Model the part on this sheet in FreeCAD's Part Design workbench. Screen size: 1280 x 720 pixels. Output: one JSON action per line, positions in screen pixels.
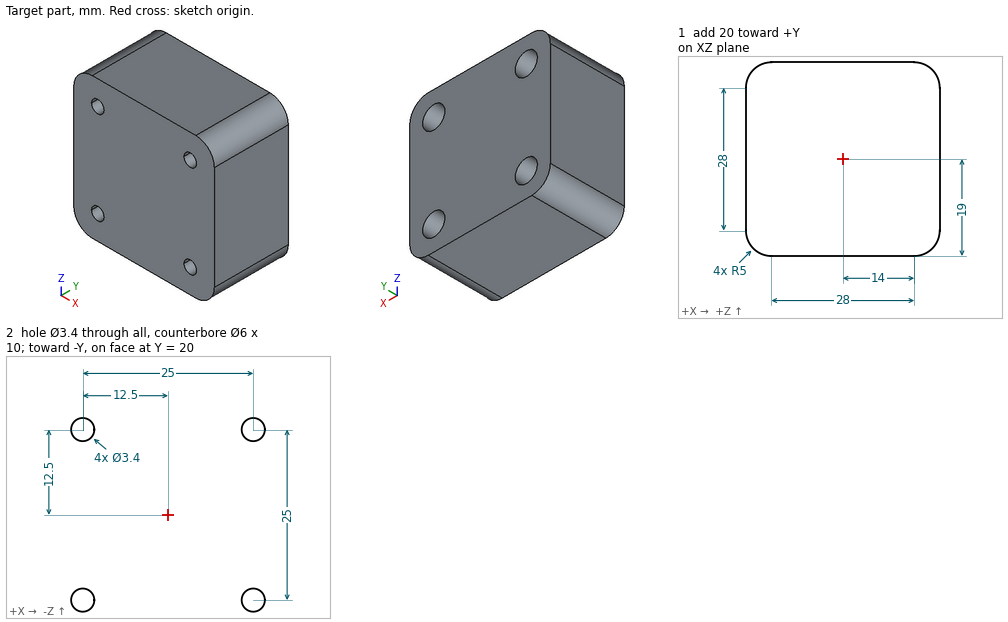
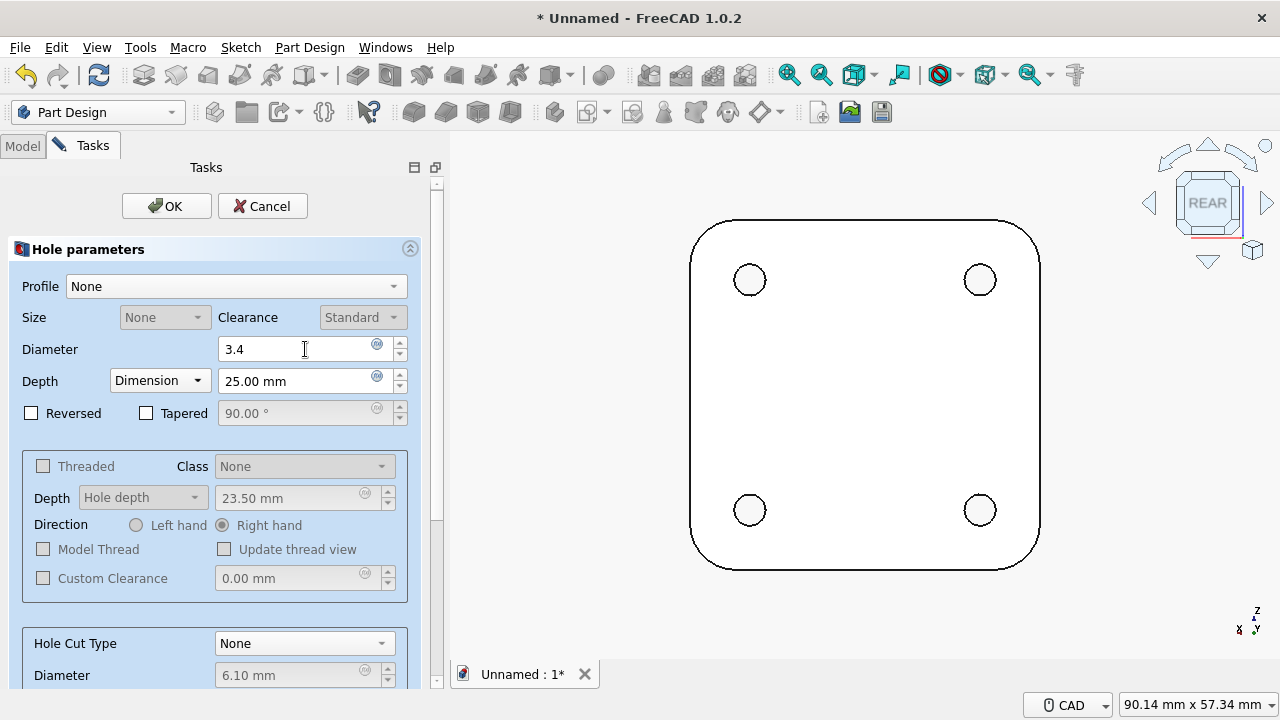
{"action": "left_click", "coordinate": [161, 380]}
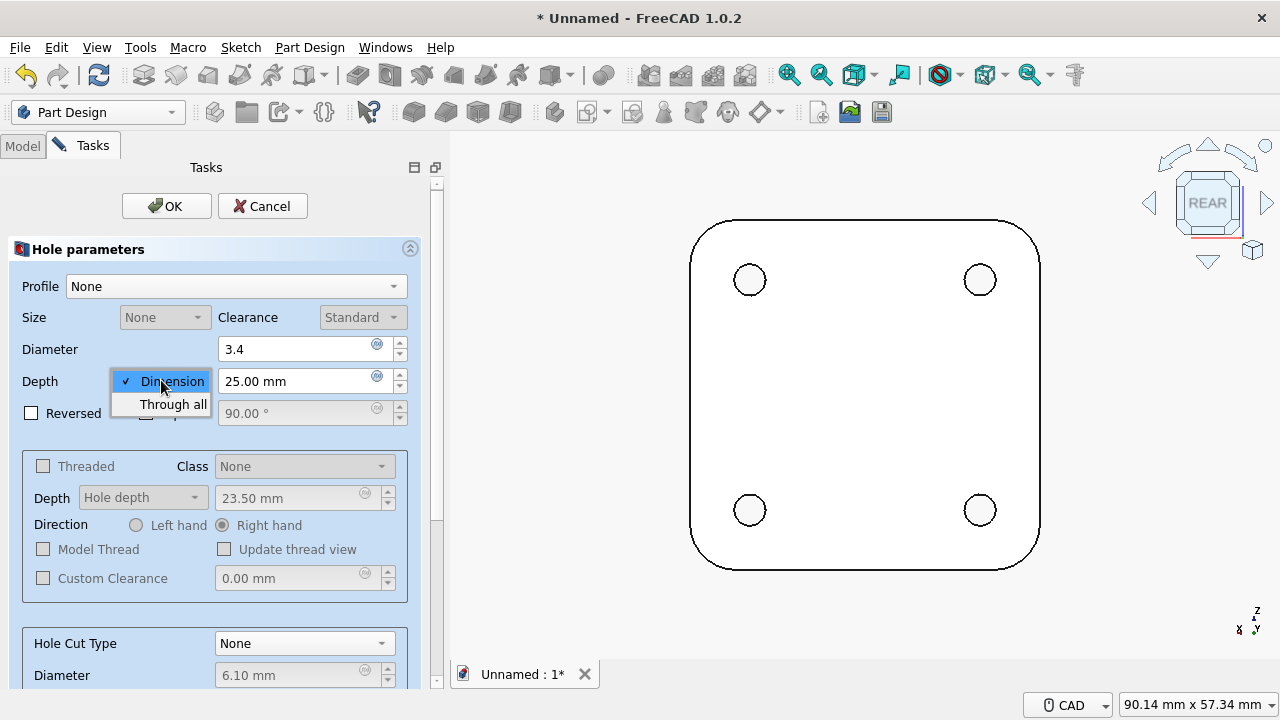
{"action": "left_click", "coordinate": [160, 404]}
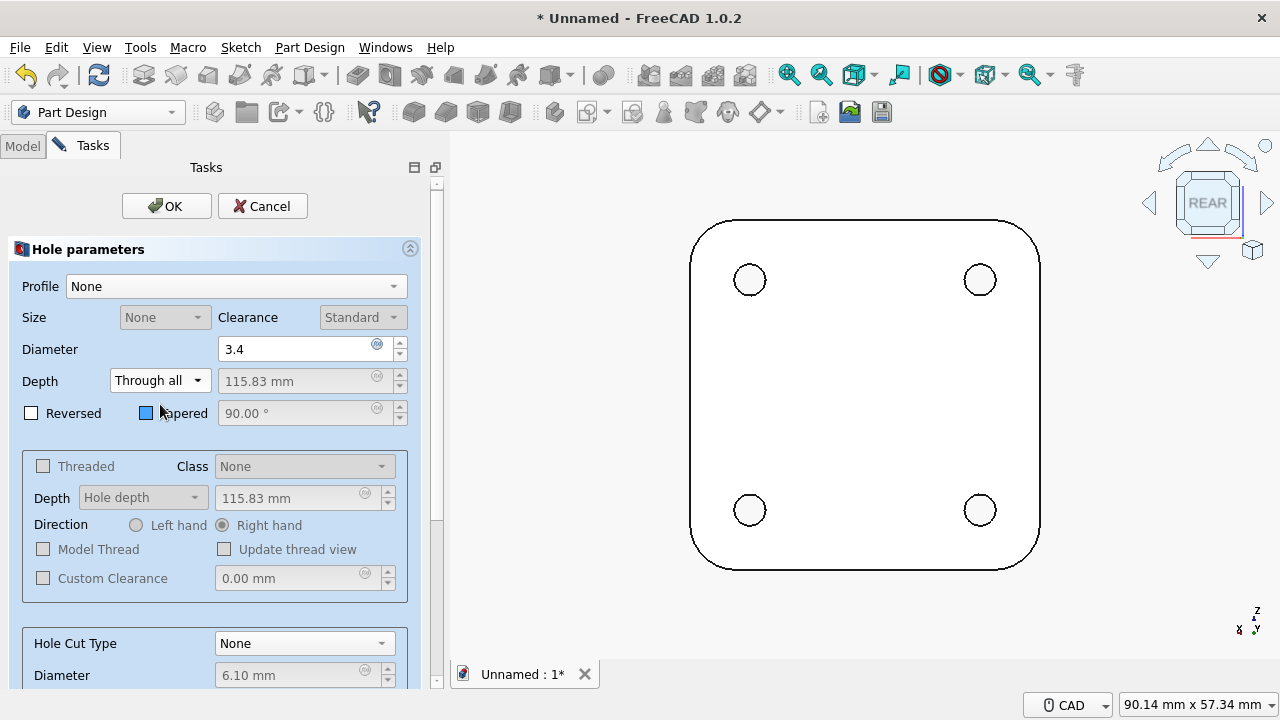
{"action": "left_click", "coordinate": [306, 644]}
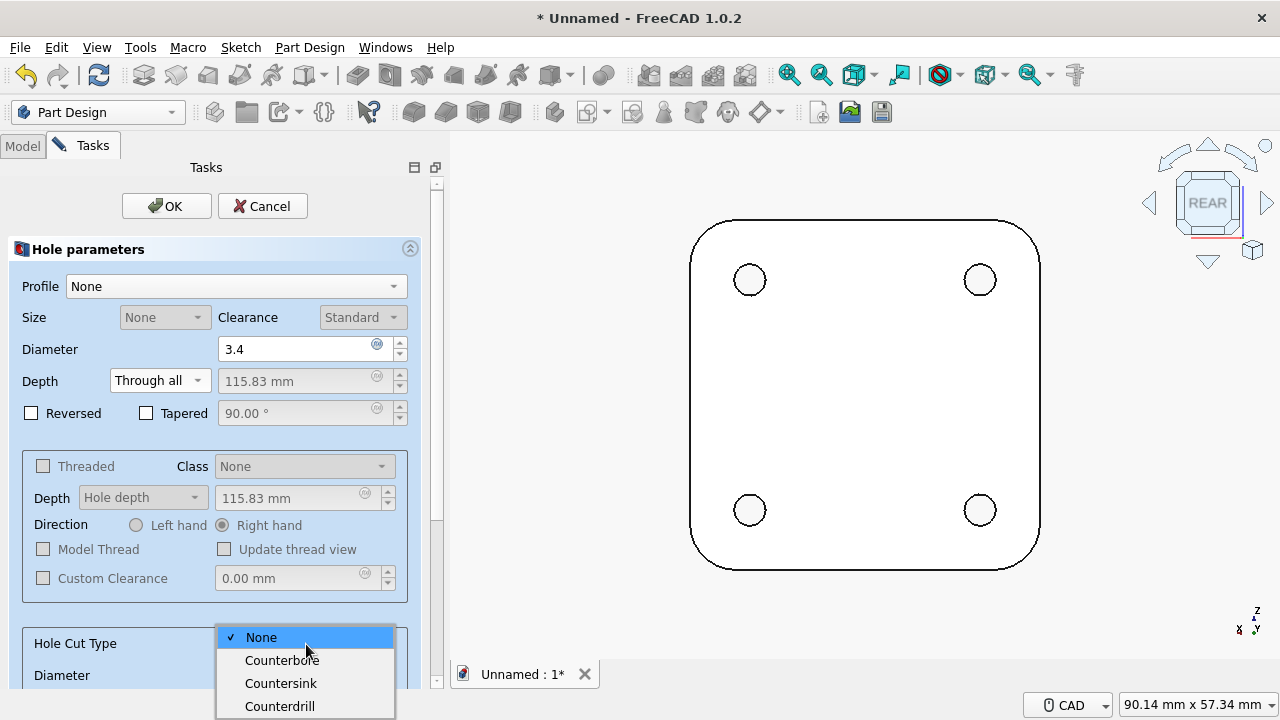
{"action": "left_click", "coordinate": [304, 660]}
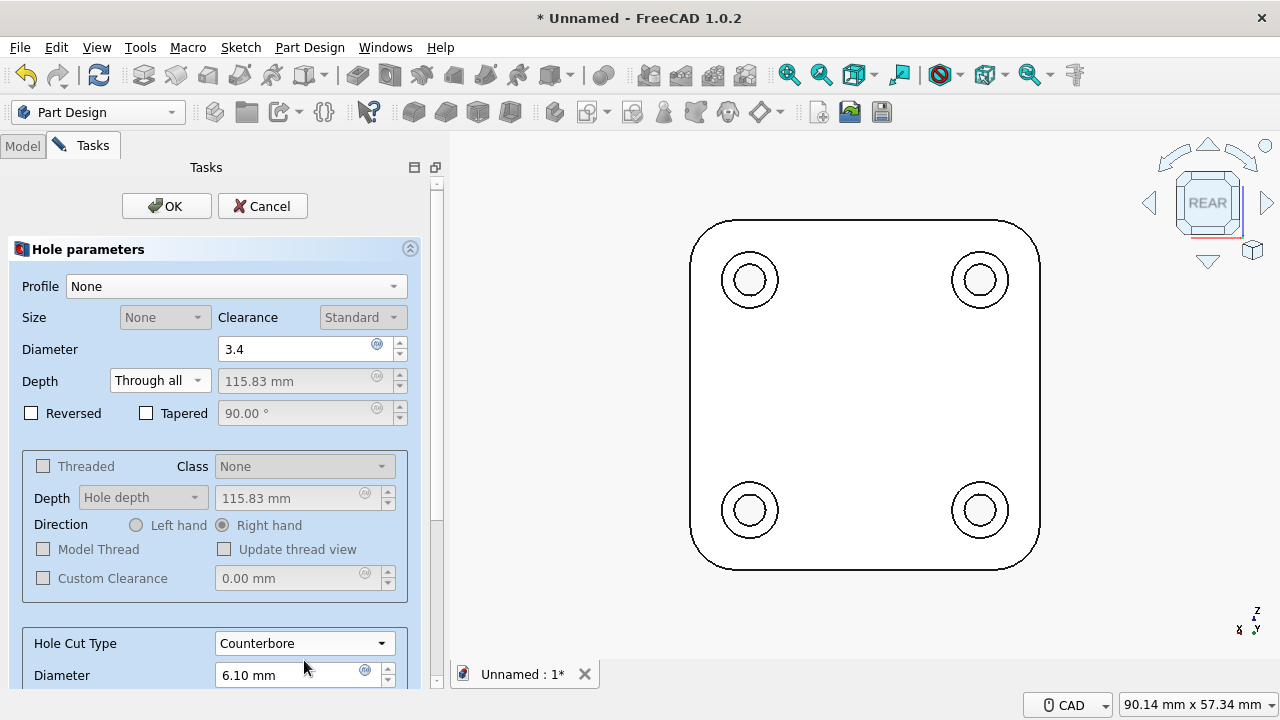
{"action": "triple_click", "coordinate": [298, 675]}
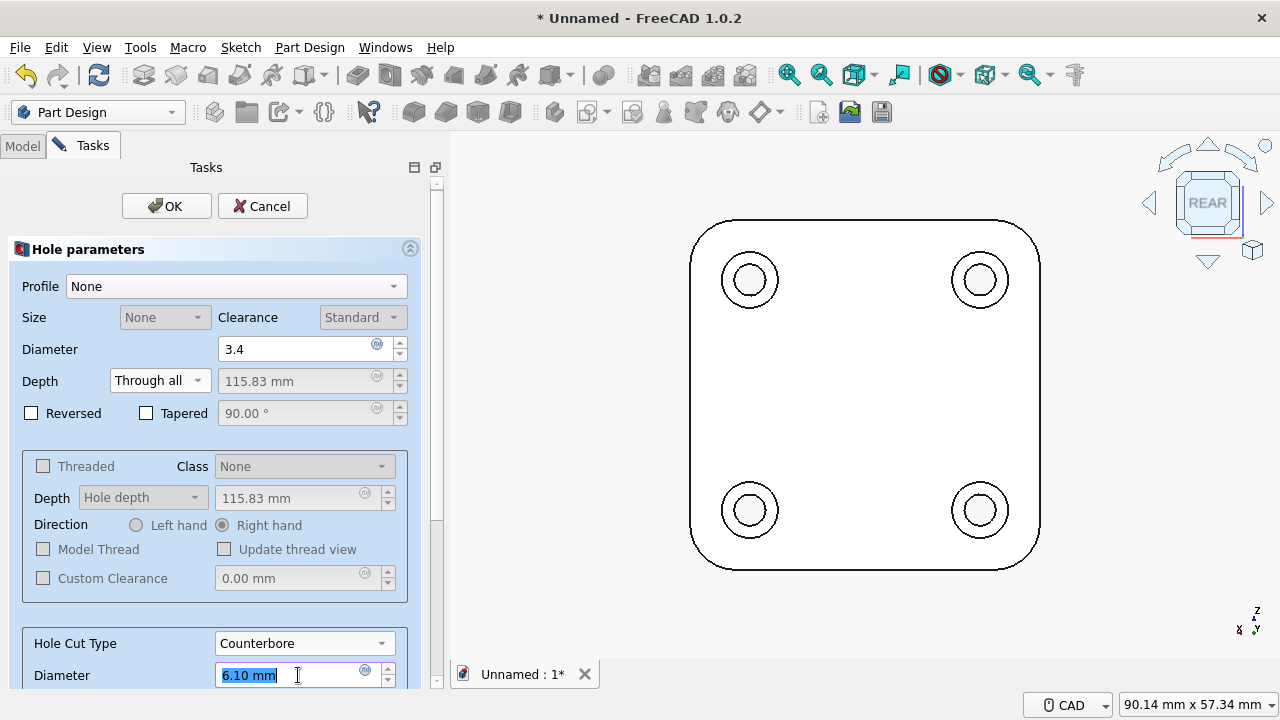
{"action": "type", "text": "6"}
{"action": "key", "text": "Tab"}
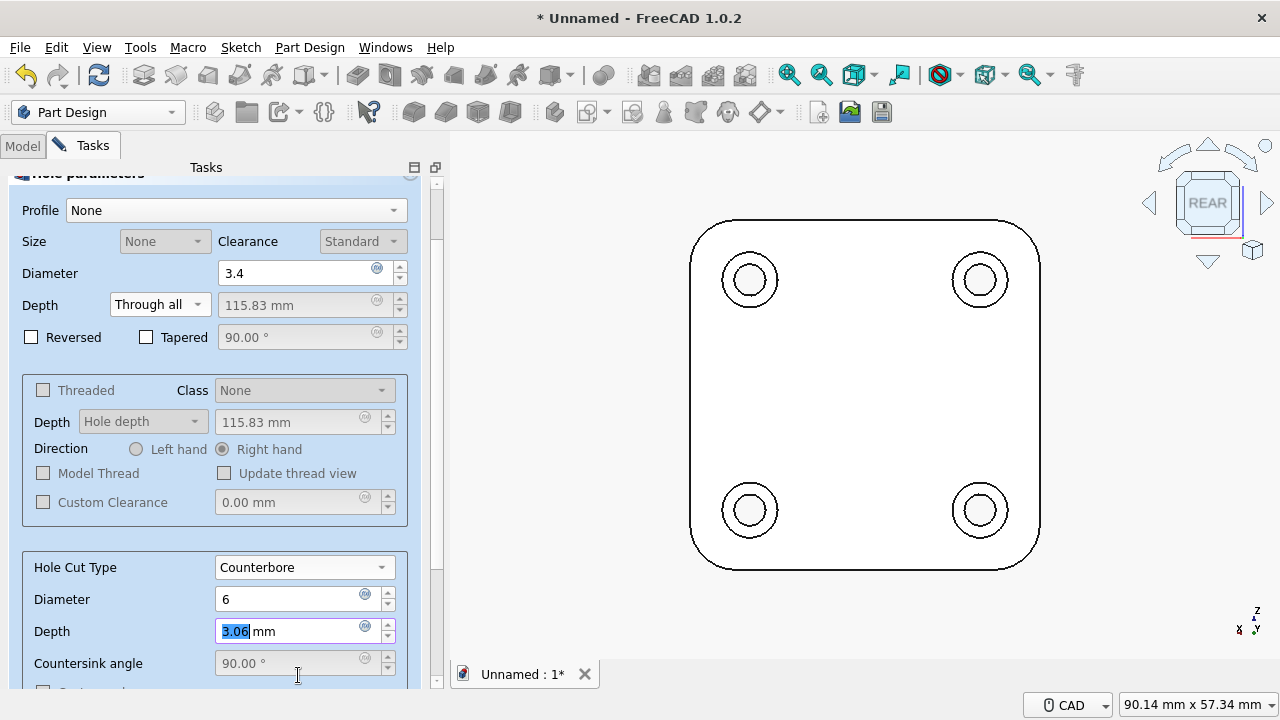
{"action": "type", "text": "10"}
{"action": "key", "text": "Tab"}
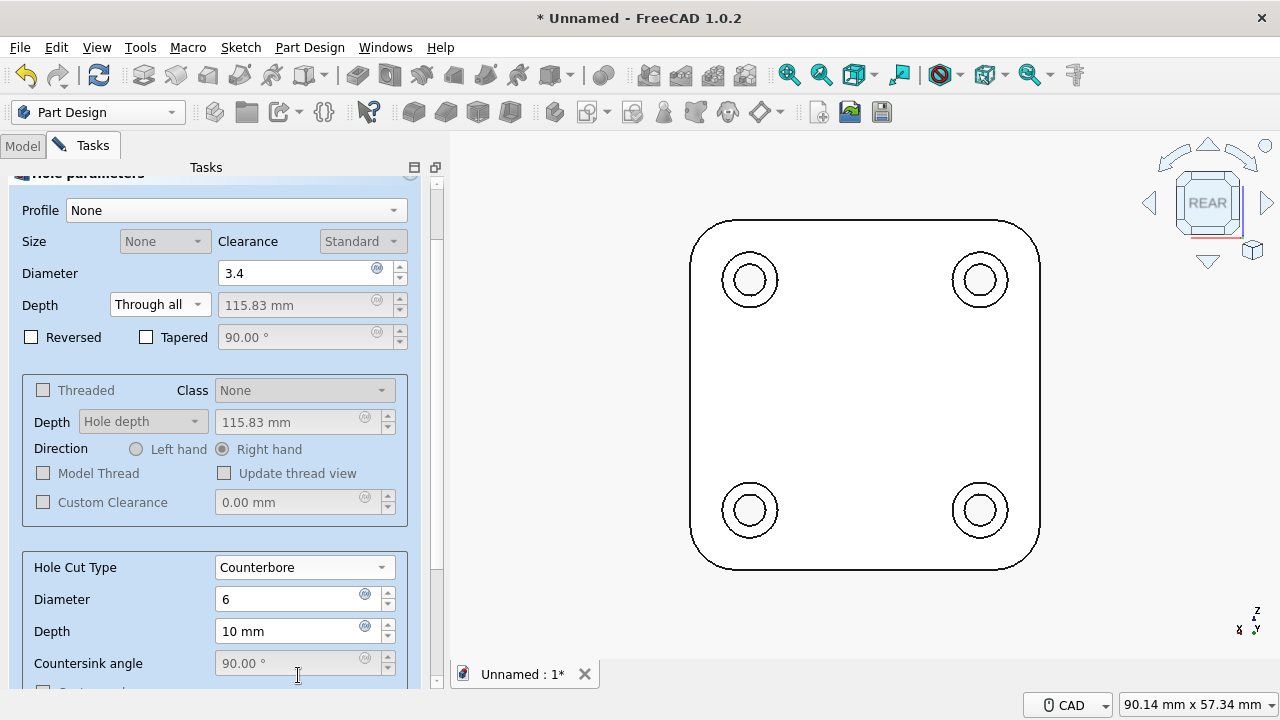
{"action": "scroll", "coordinate": [437, 432], "scroll_direction": "up", "scroll_amount": 3}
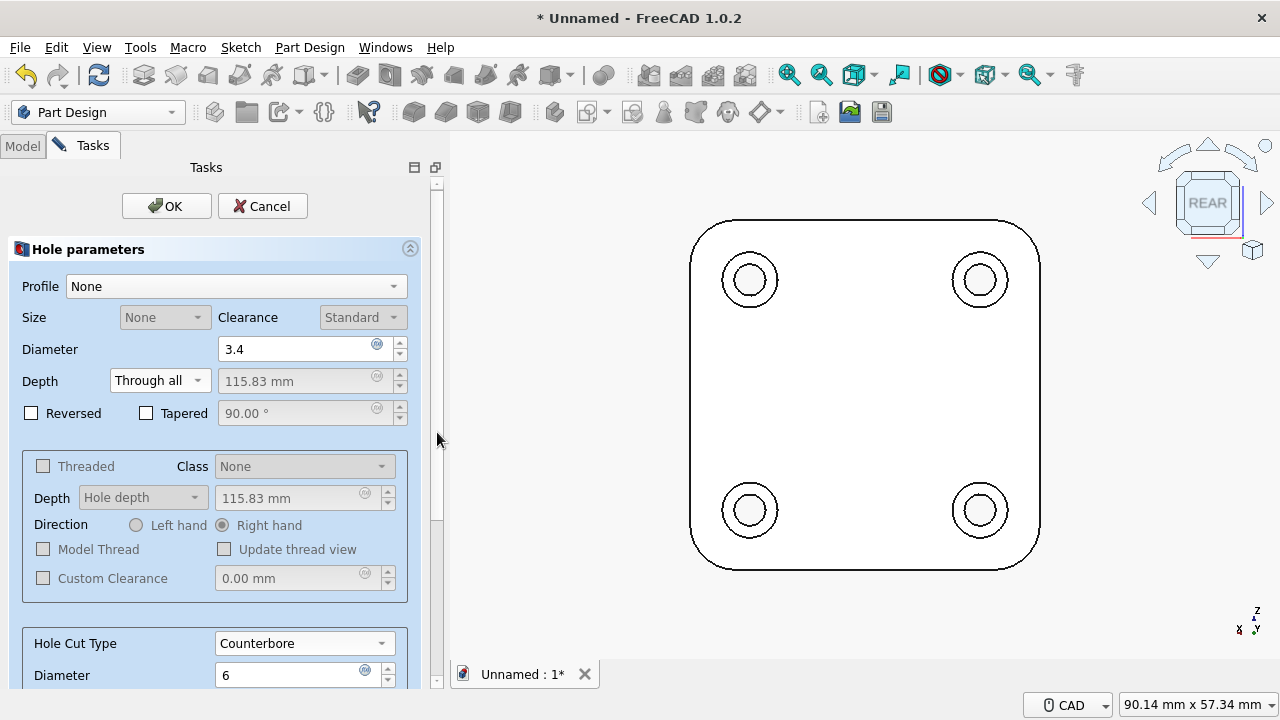
{"action": "left_click", "coordinate": [167, 206]}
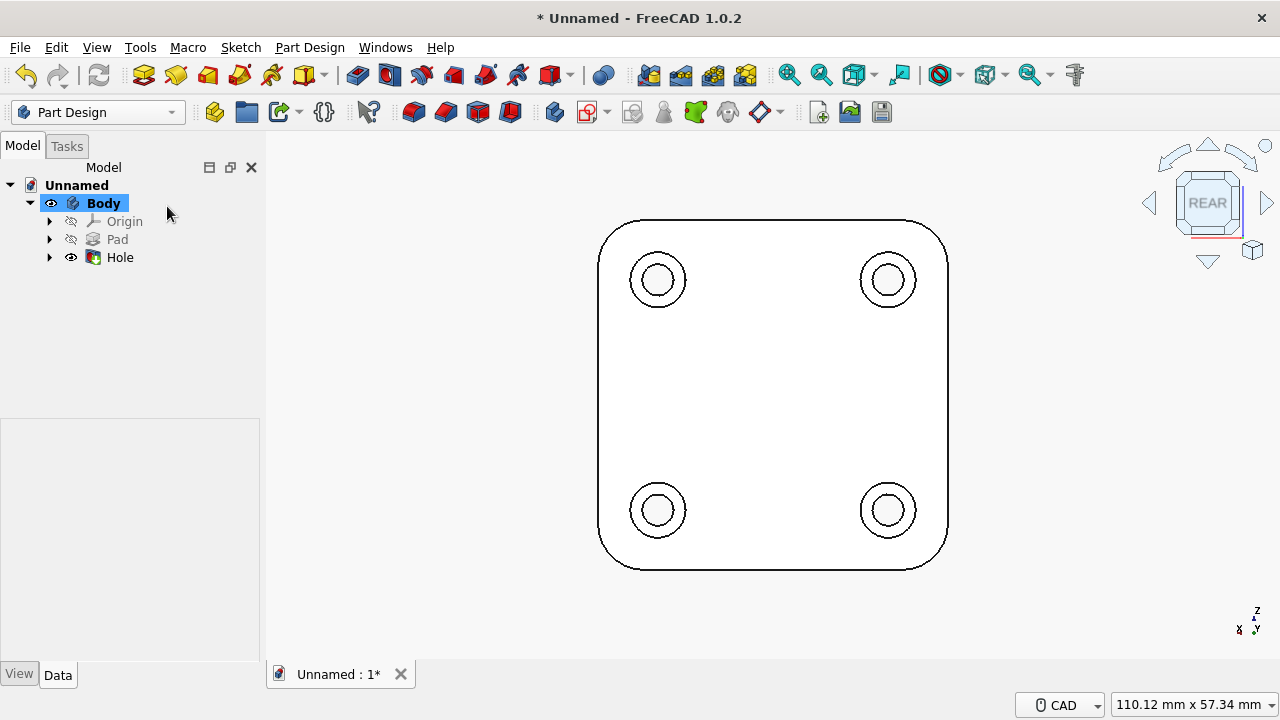
{"action": "key", "text": "0"}